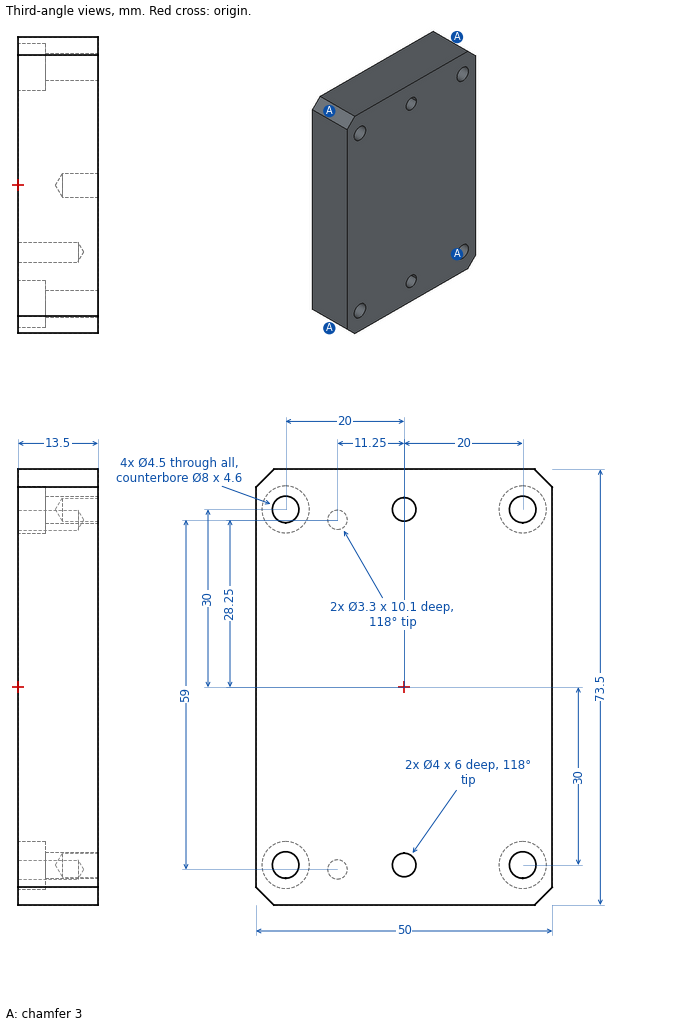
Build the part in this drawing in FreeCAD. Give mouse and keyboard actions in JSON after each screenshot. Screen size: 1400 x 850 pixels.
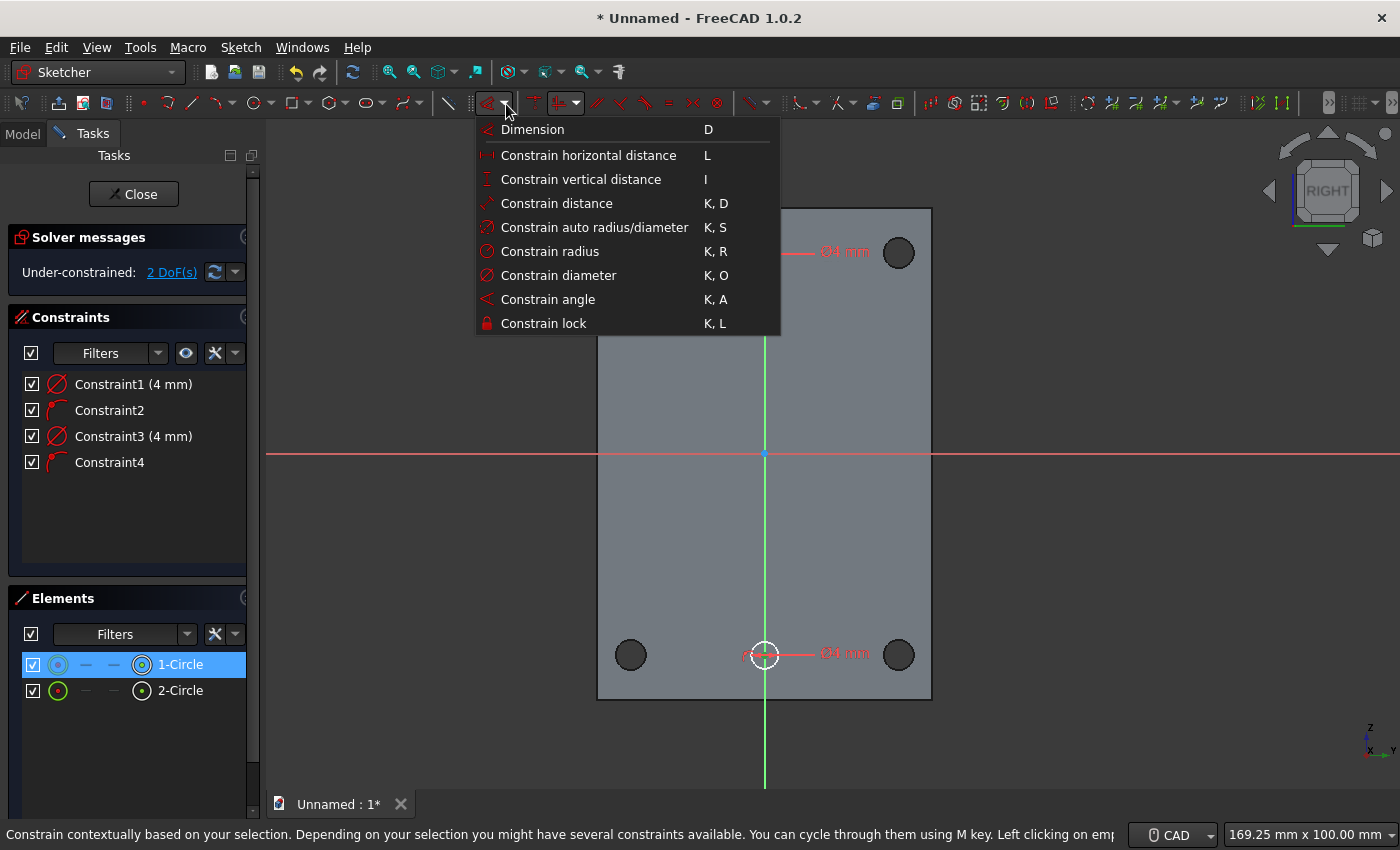
{"action": "left_click", "coordinate": [628, 179]}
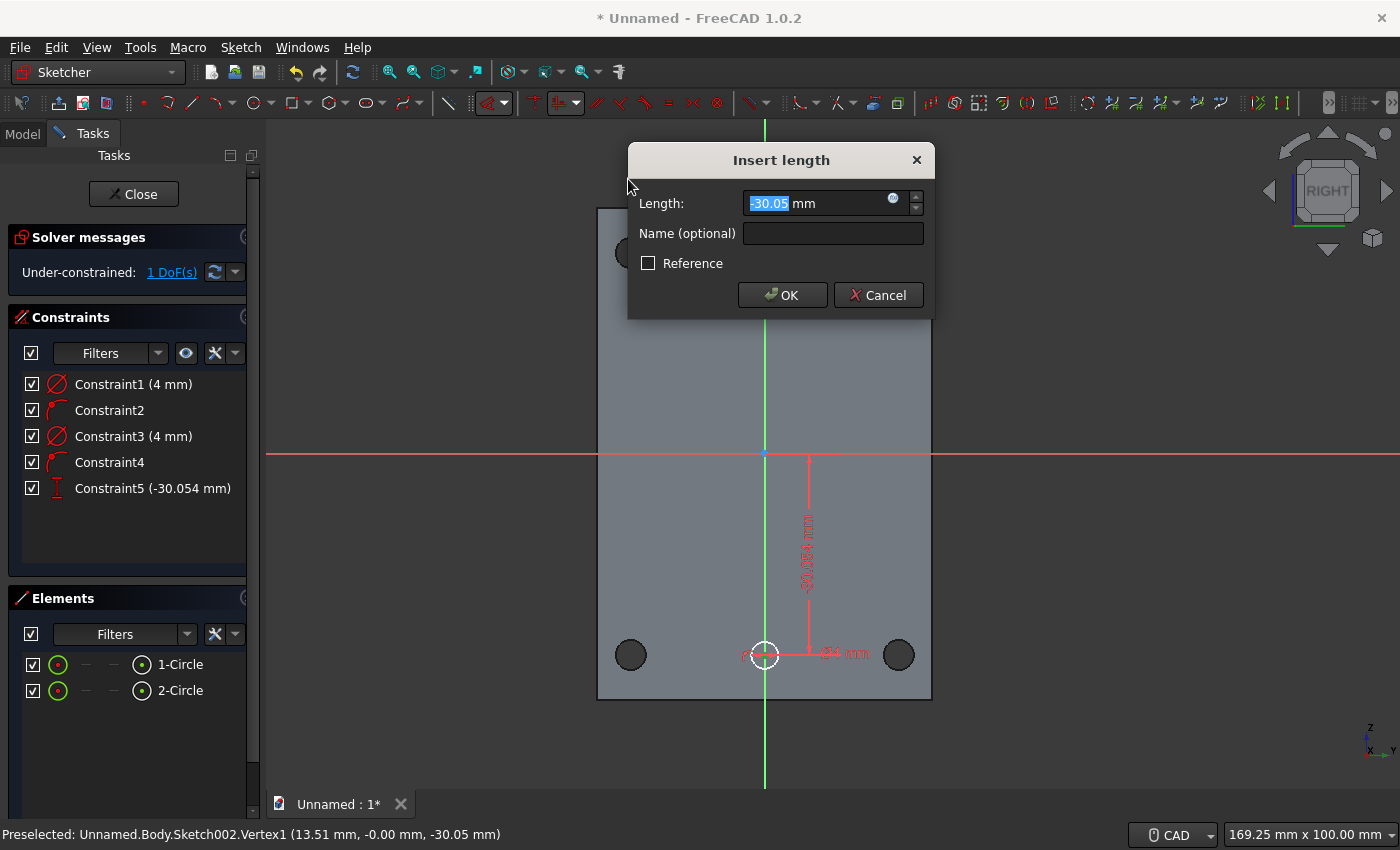
{"action": "type", "text": "-30"}
{"action": "key", "text": "Return"}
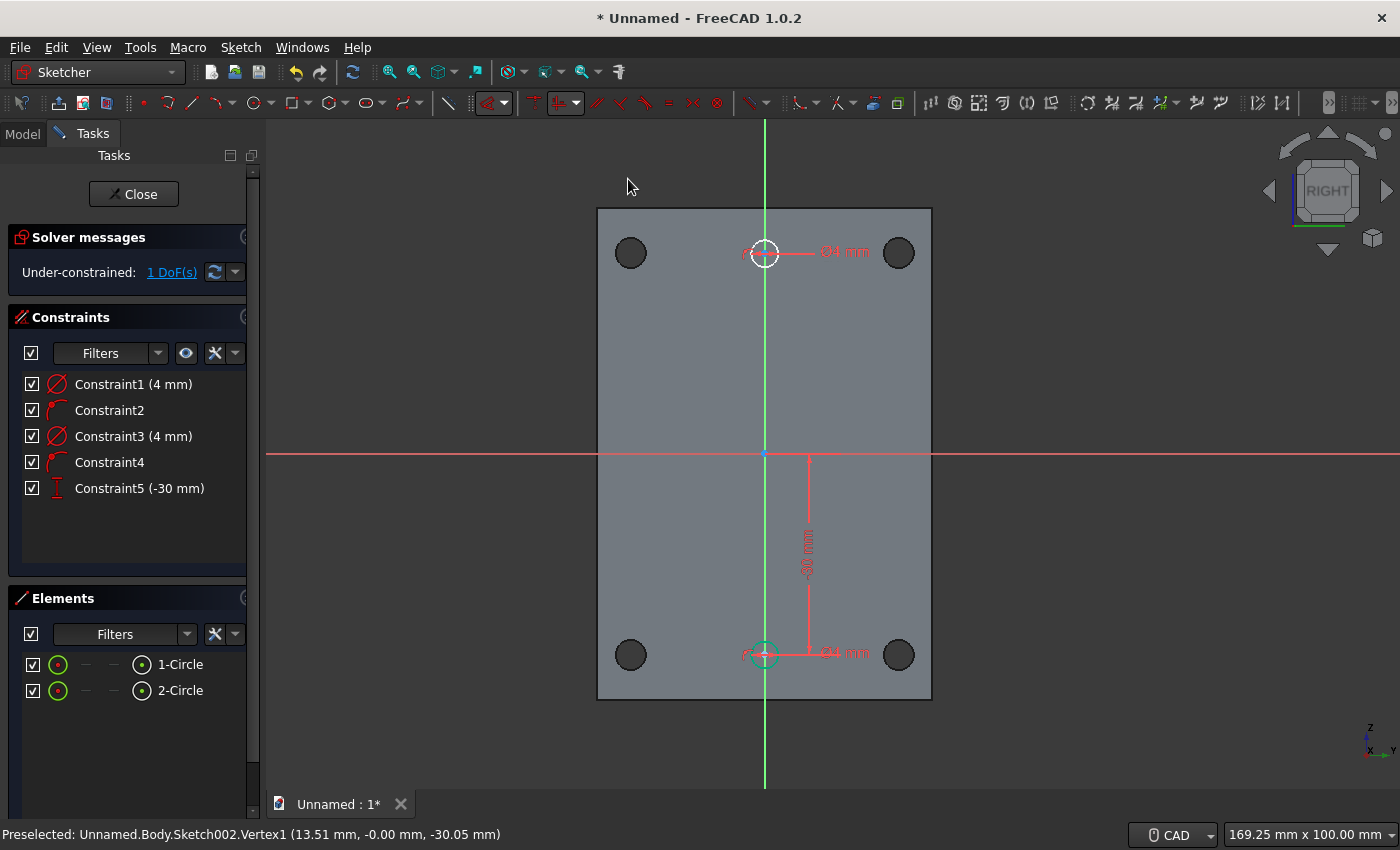
{"action": "left_click", "coordinate": [765, 254]}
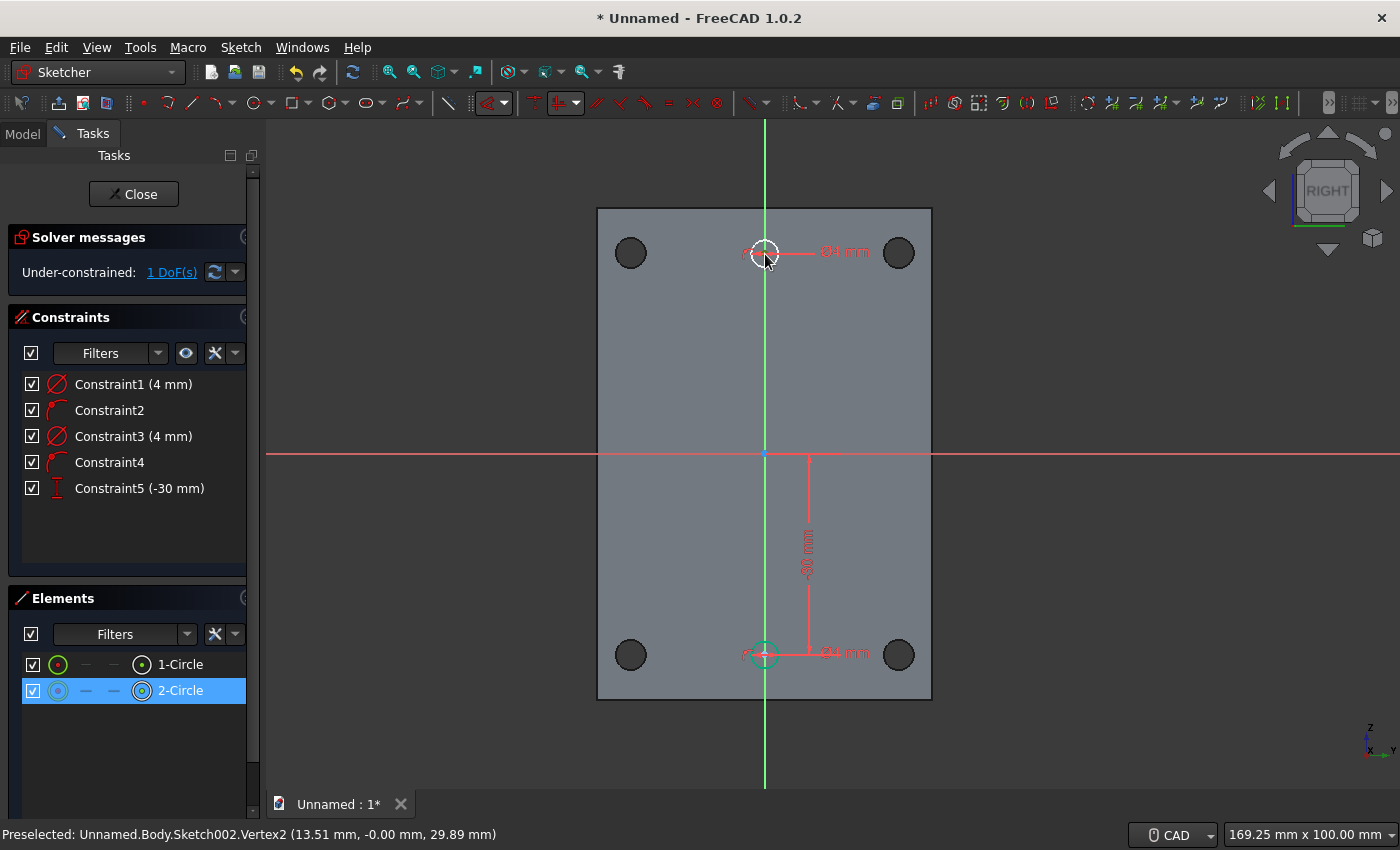
{"action": "left_click", "coordinate": [506, 104]}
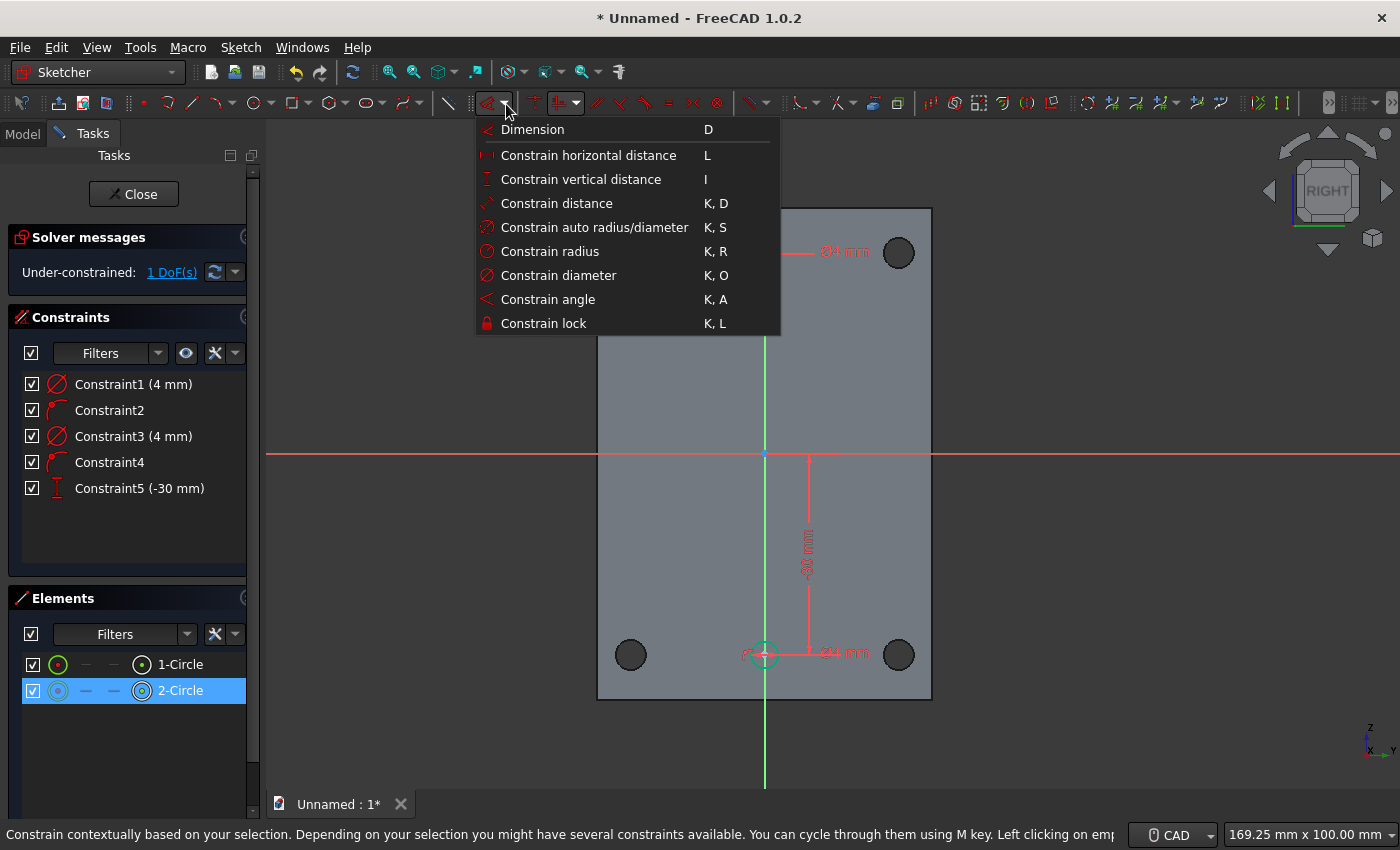
{"action": "left_click", "coordinate": [628, 179]}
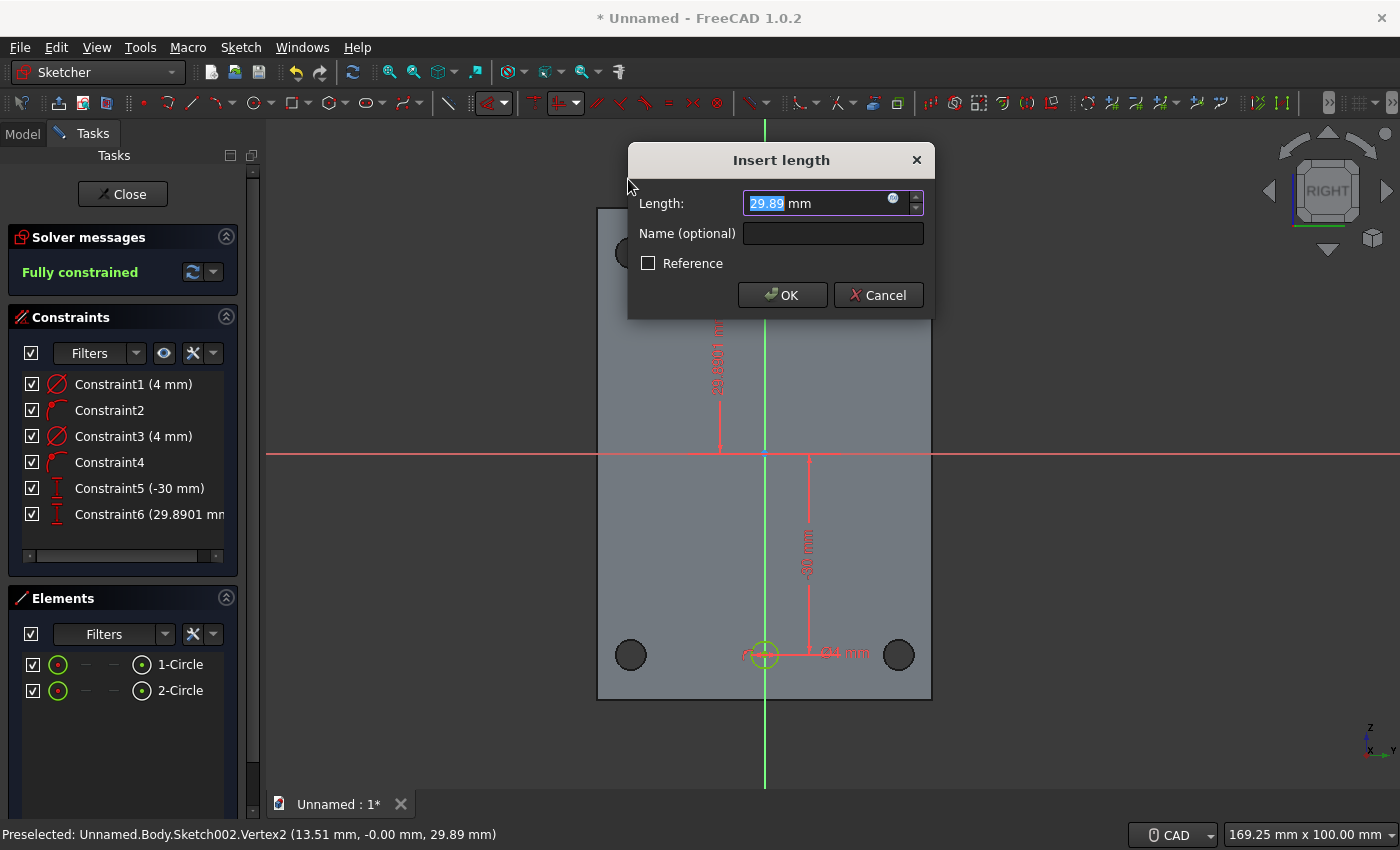
{"action": "type", "text": "30"}
{"action": "key", "text": "Return"}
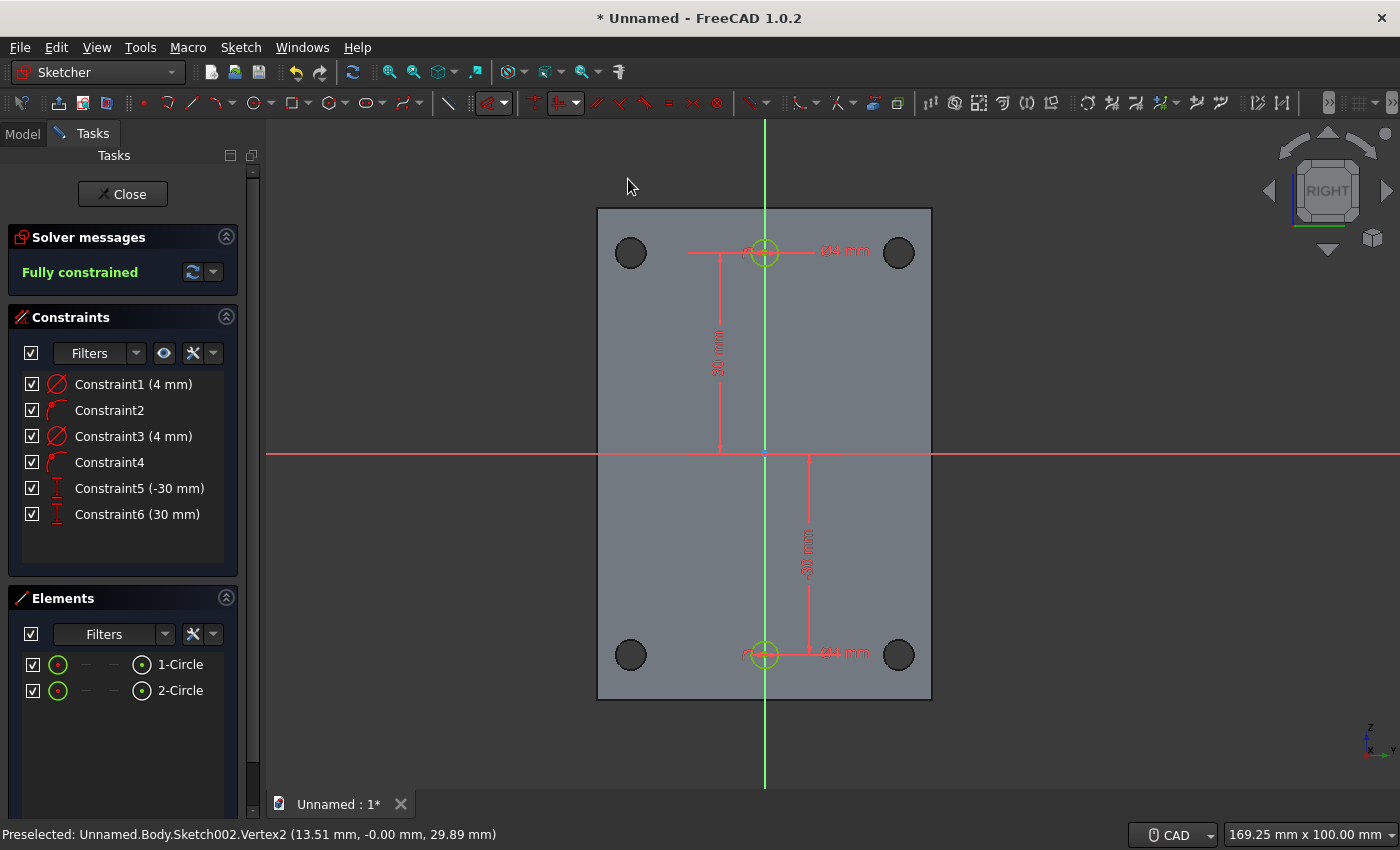
{"action": "left_click", "coordinate": [123, 194]}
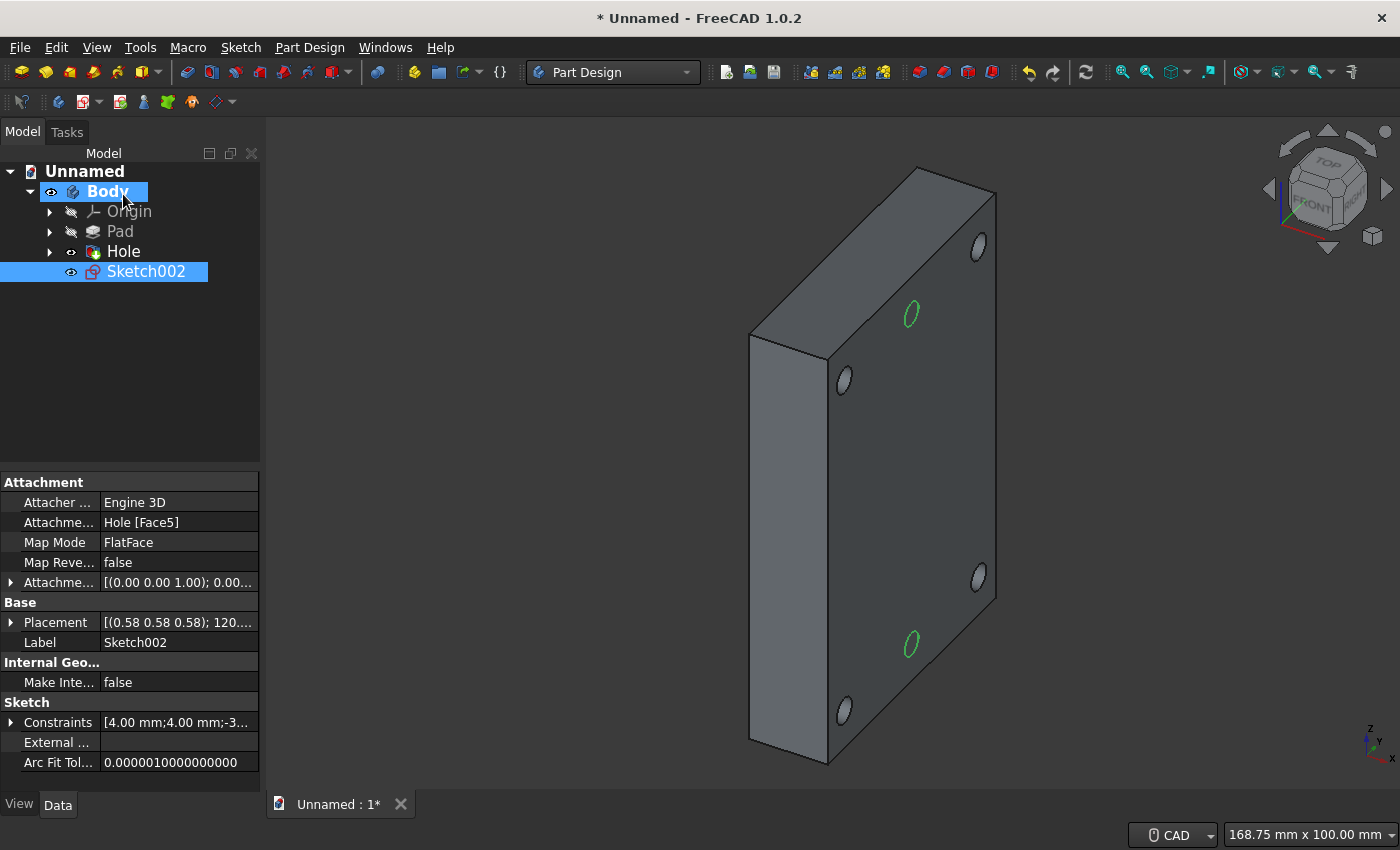
{"action": "left_click", "coordinate": [212, 72]}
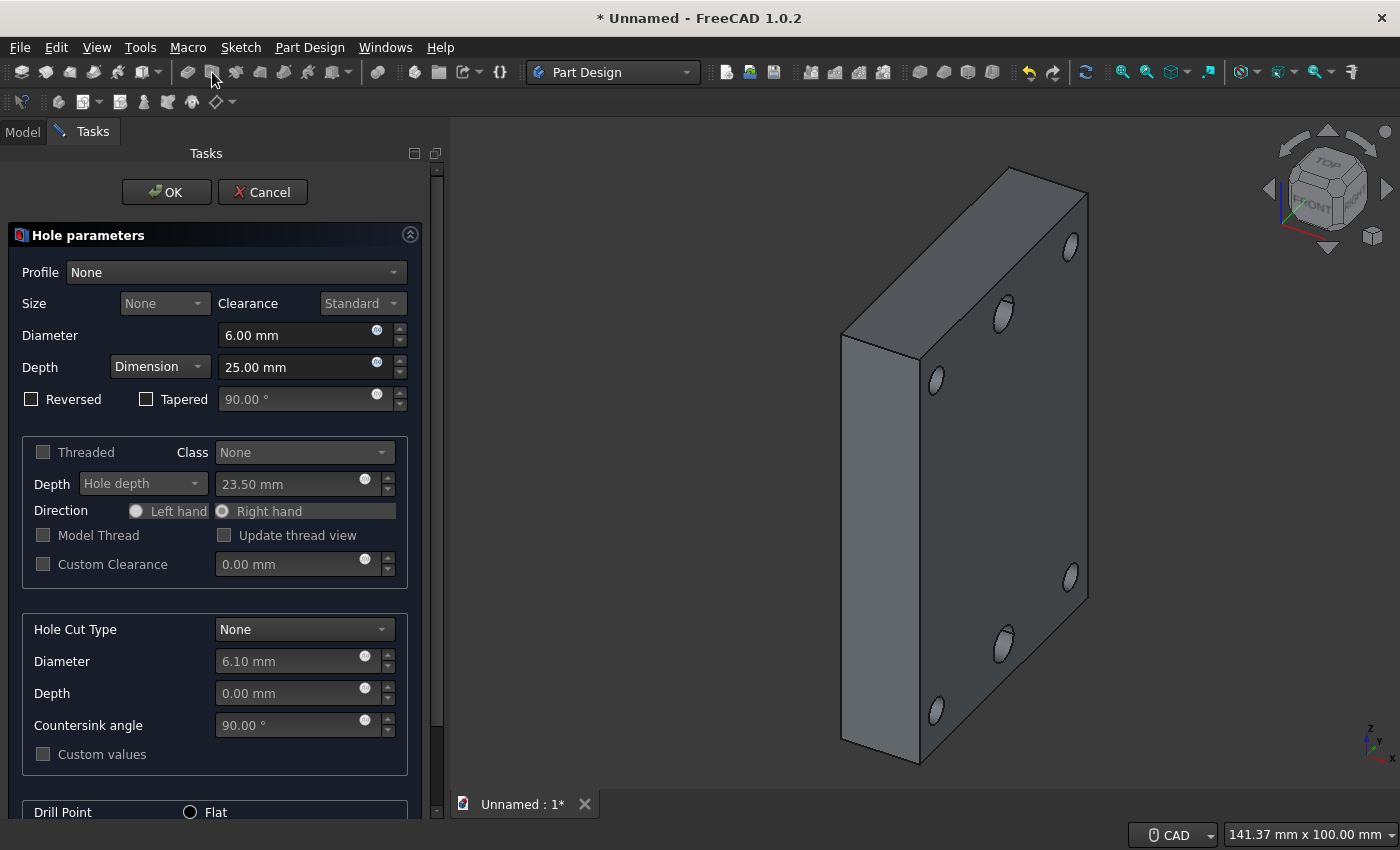
{"action": "triple_click", "coordinate": [305, 335]}